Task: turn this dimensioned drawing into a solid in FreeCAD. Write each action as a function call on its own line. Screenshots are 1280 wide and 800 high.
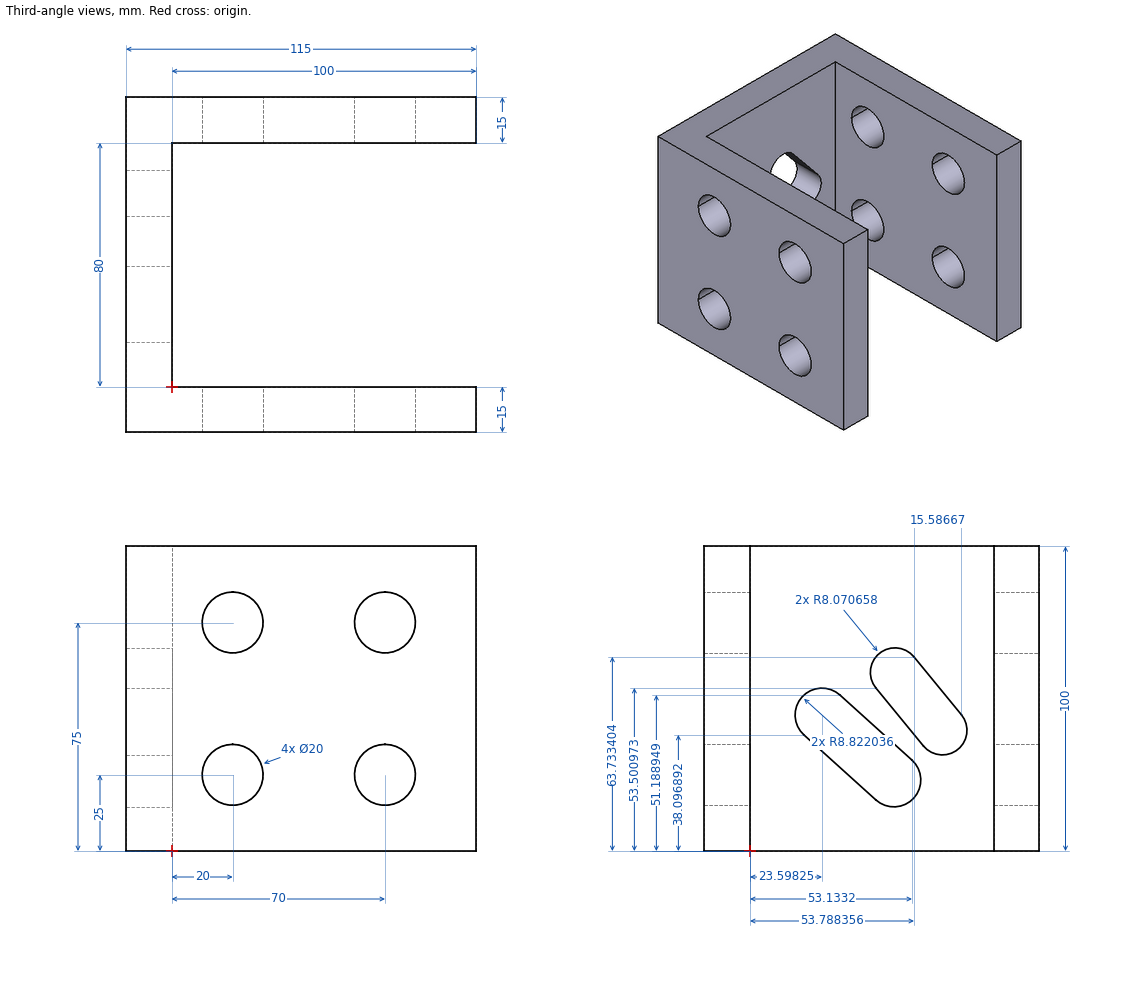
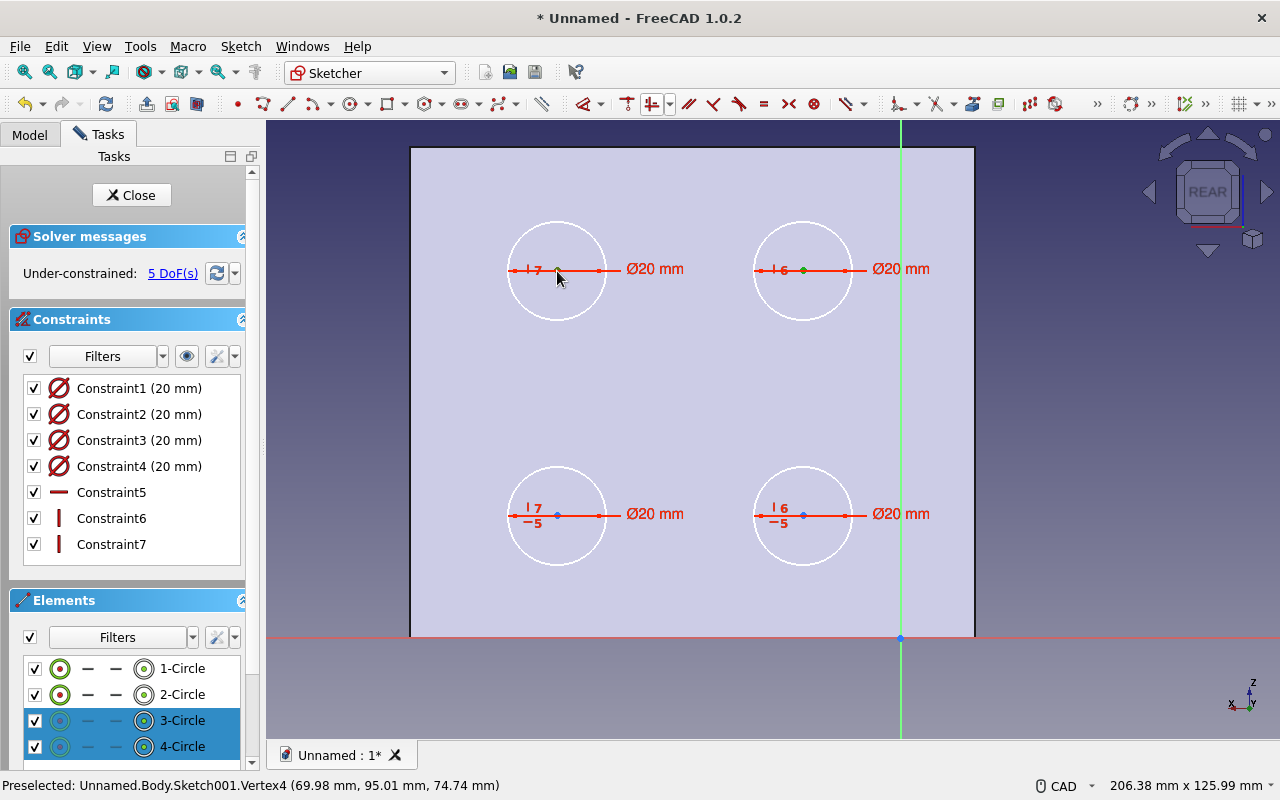
click(670, 104)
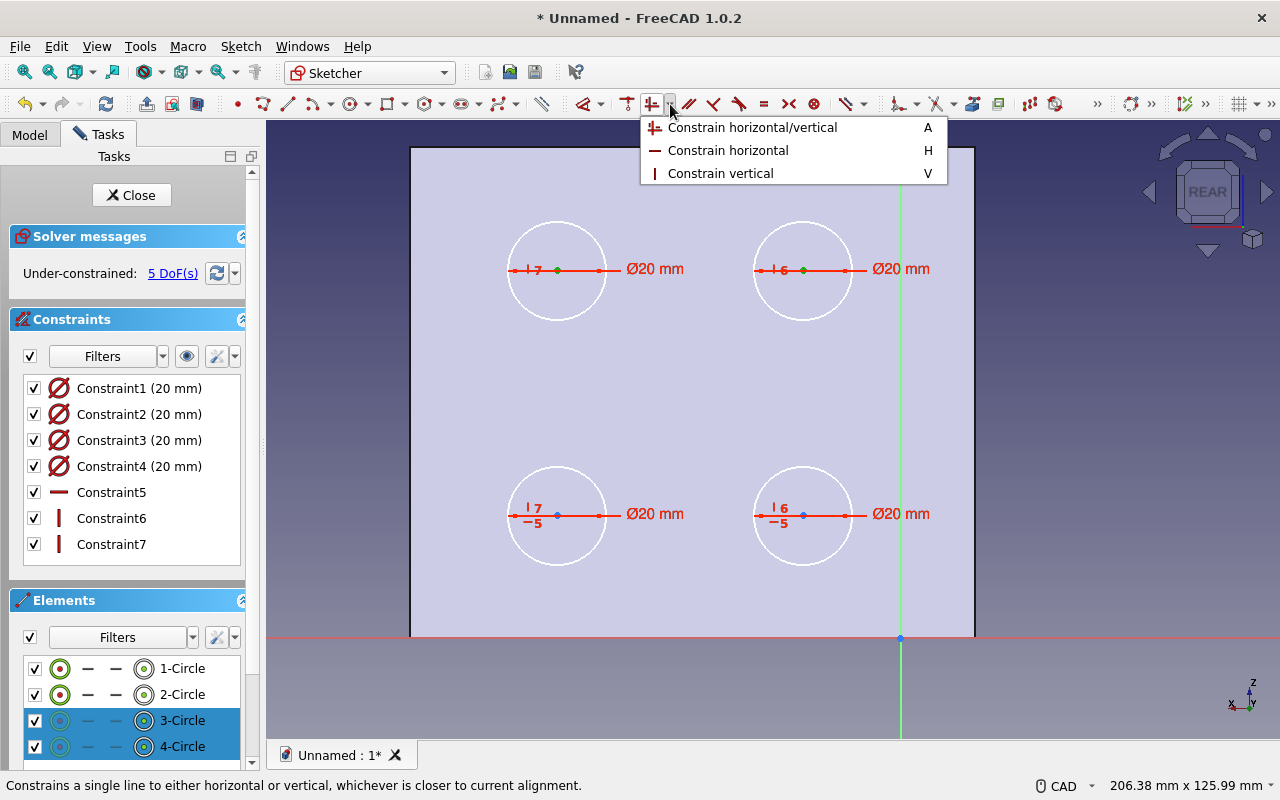
click(794, 150)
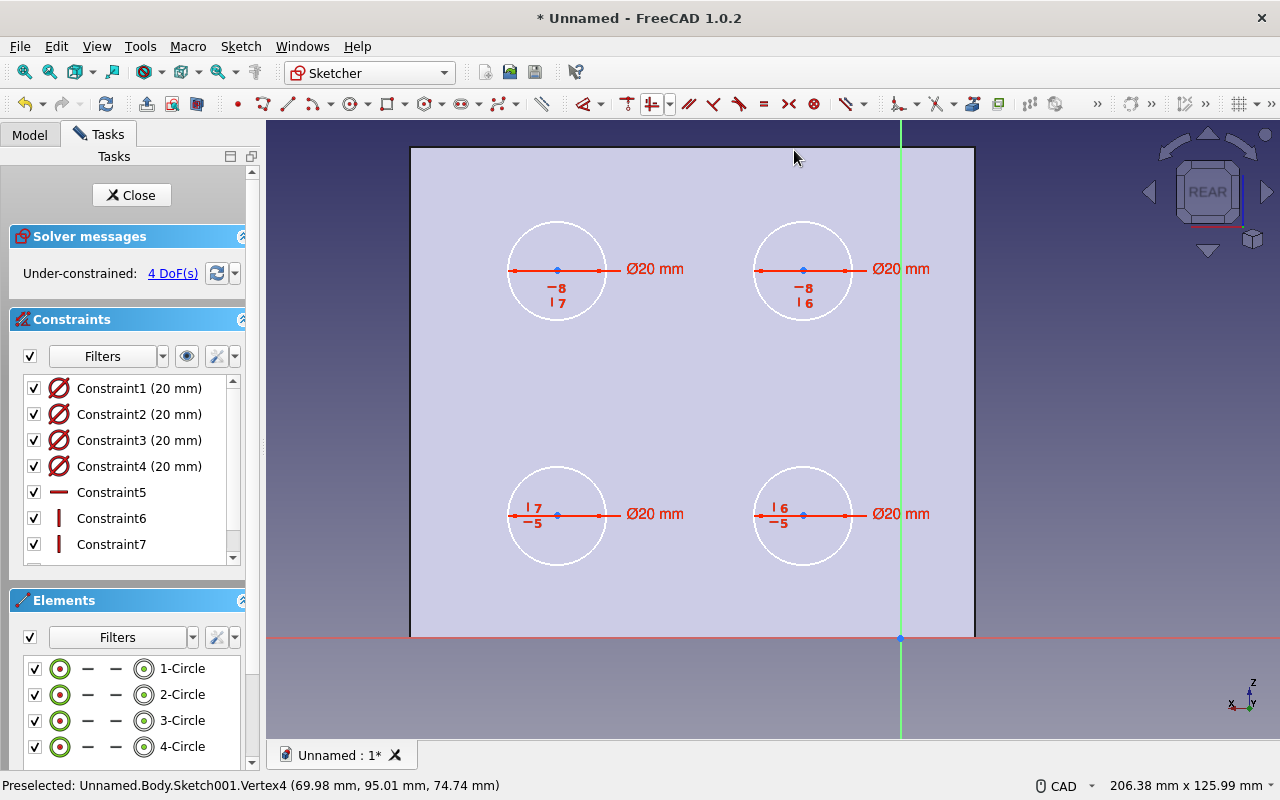
click(582, 104)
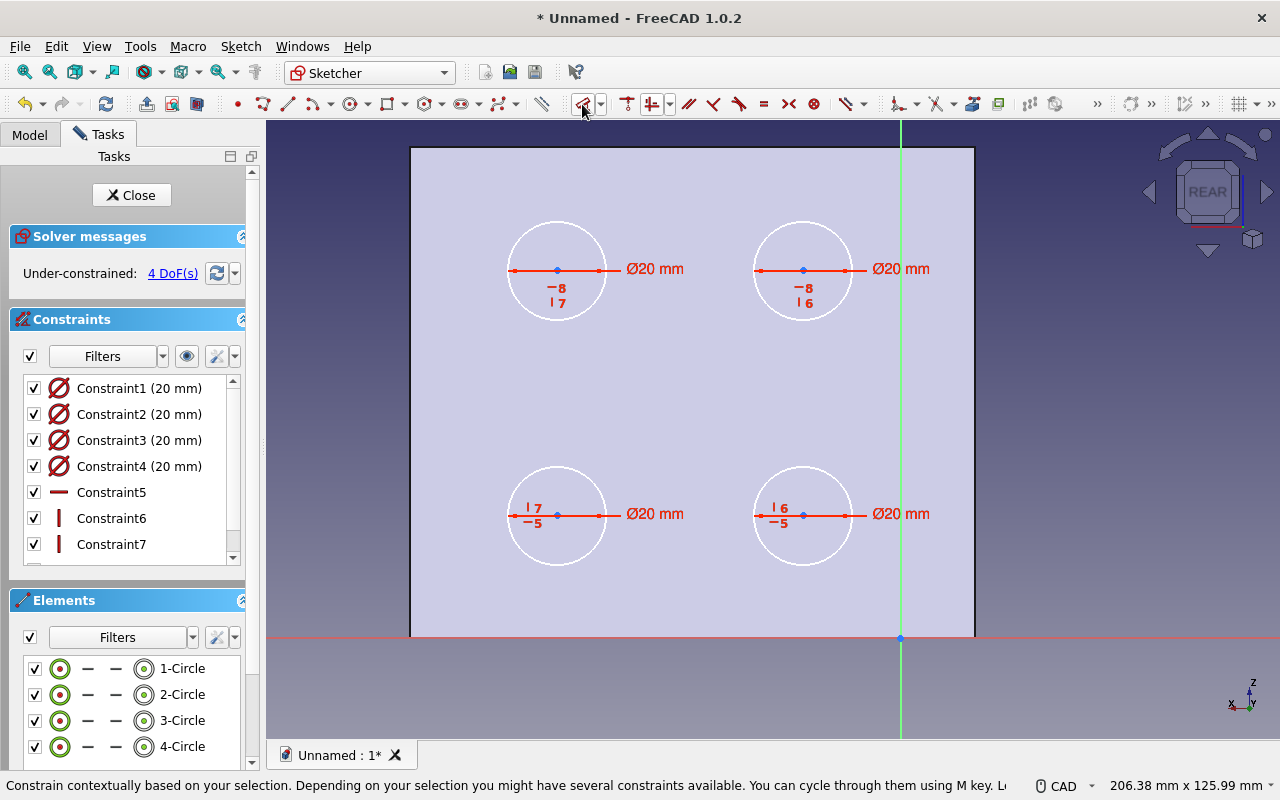
click(803, 516)
click(852, 672)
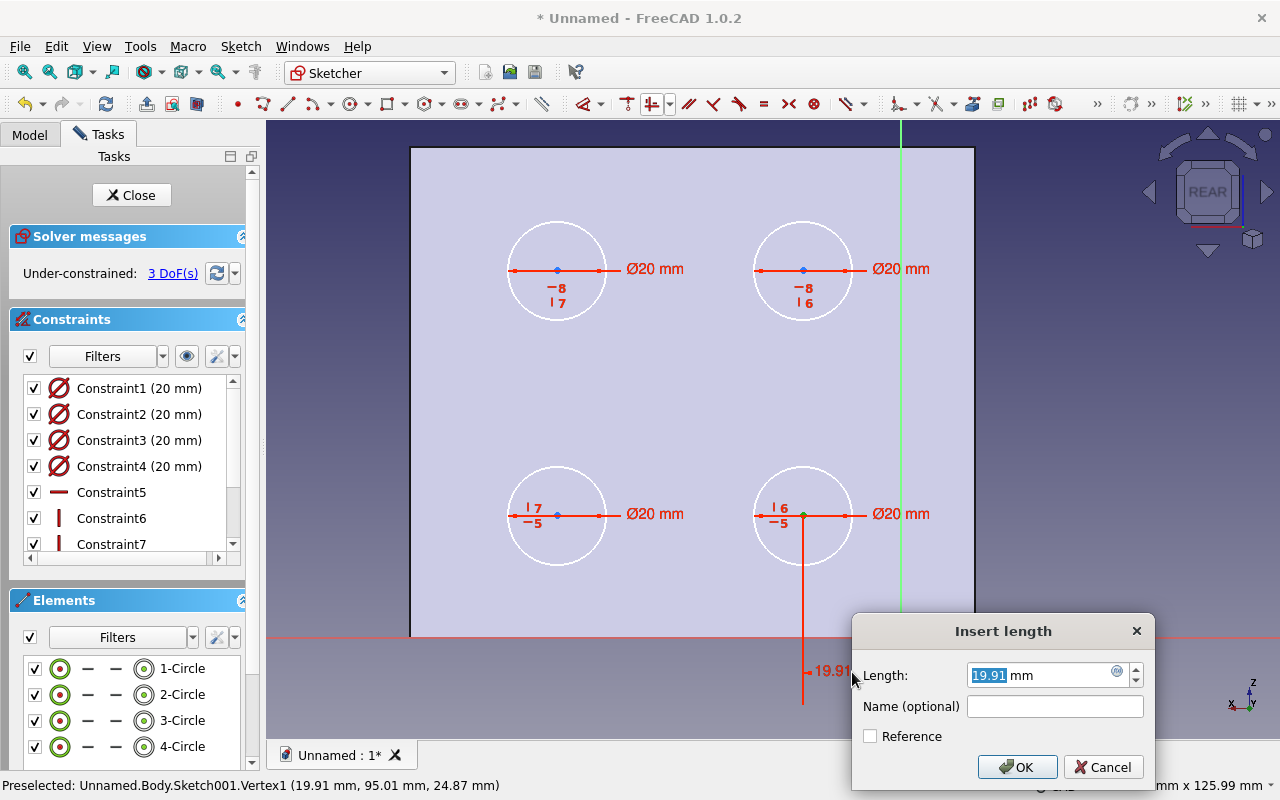
text(20)
key(Return)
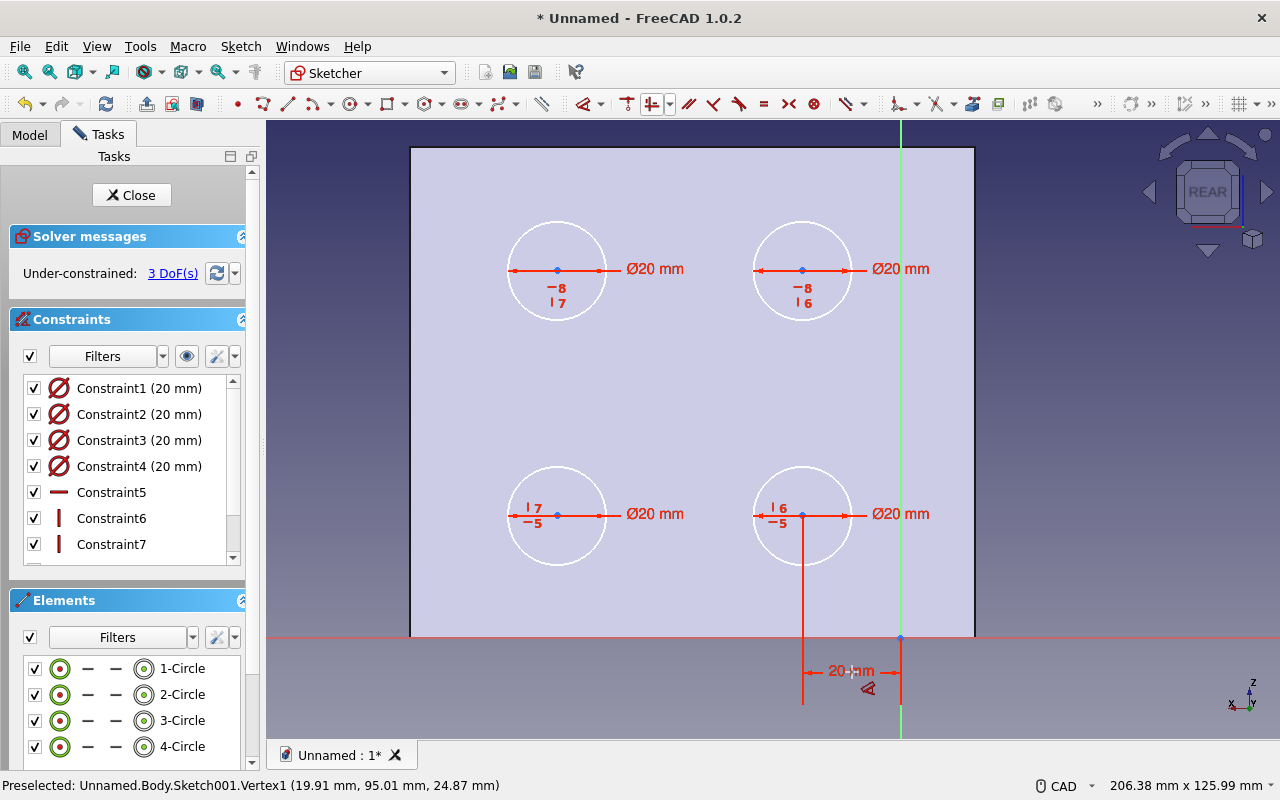
click(803, 516)
click(935, 577)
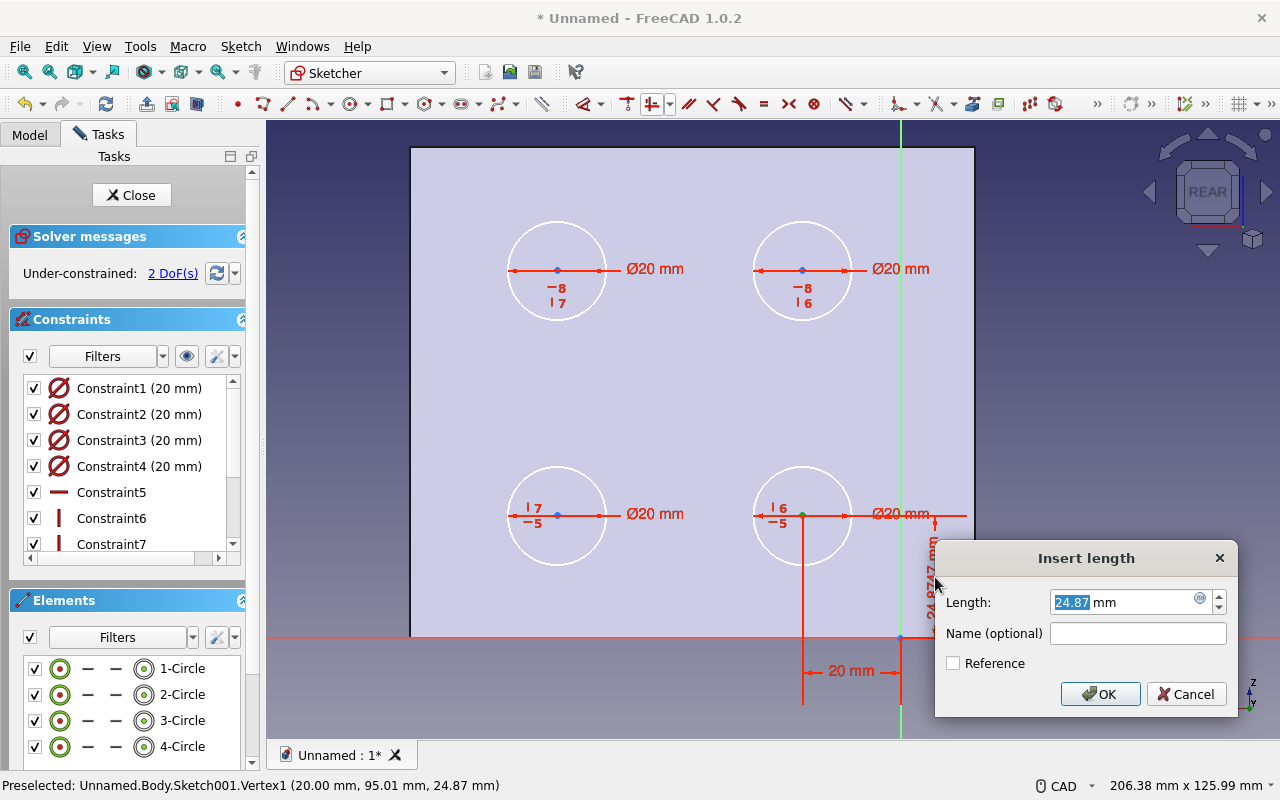
text(25)
key(Return)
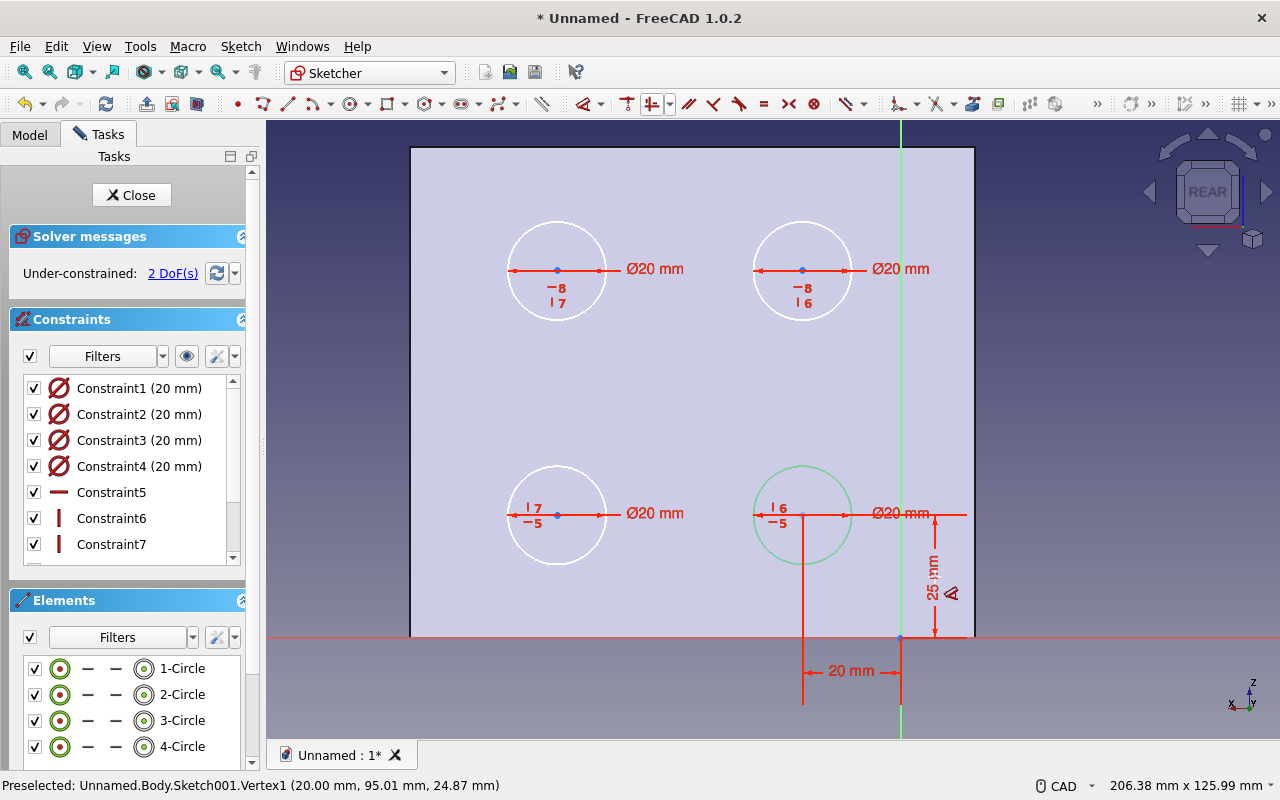
click(557, 515)
click(729, 672)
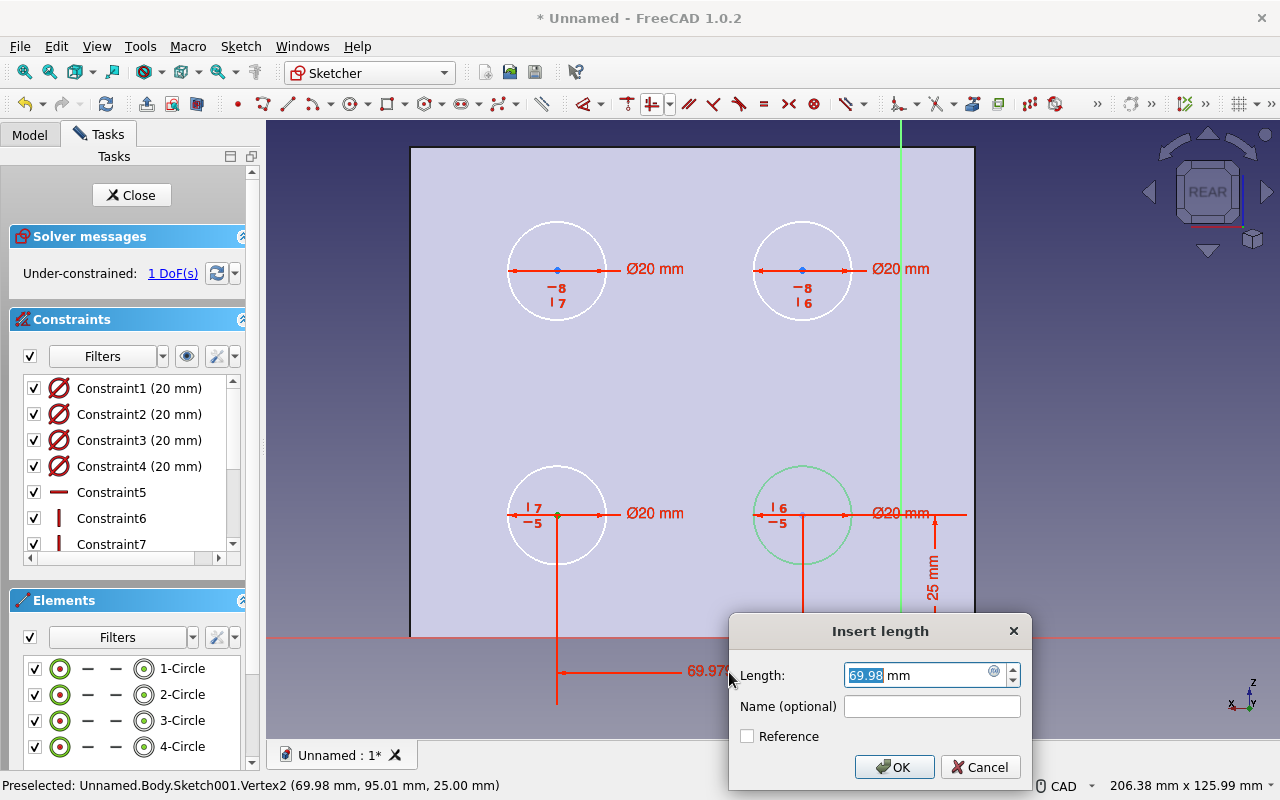
text(70)
key(Return)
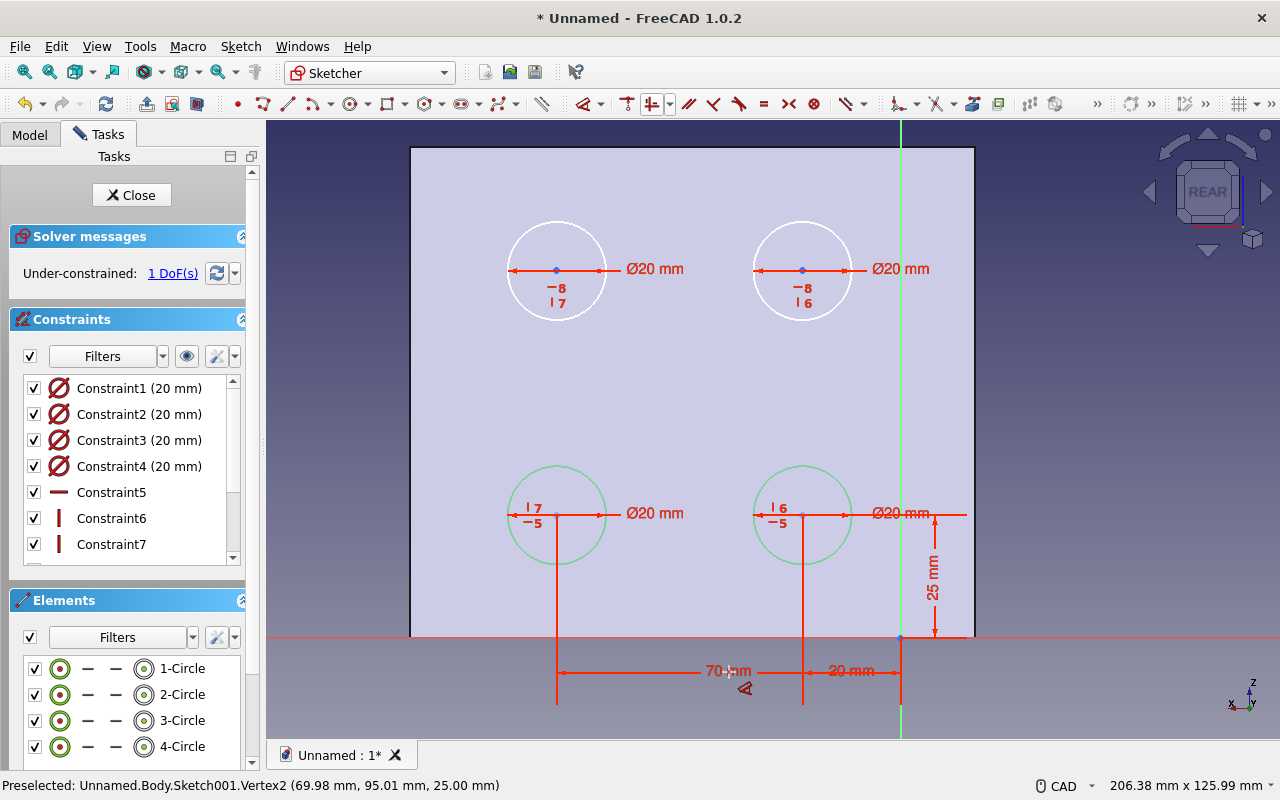
click(803, 271)
click(935, 455)